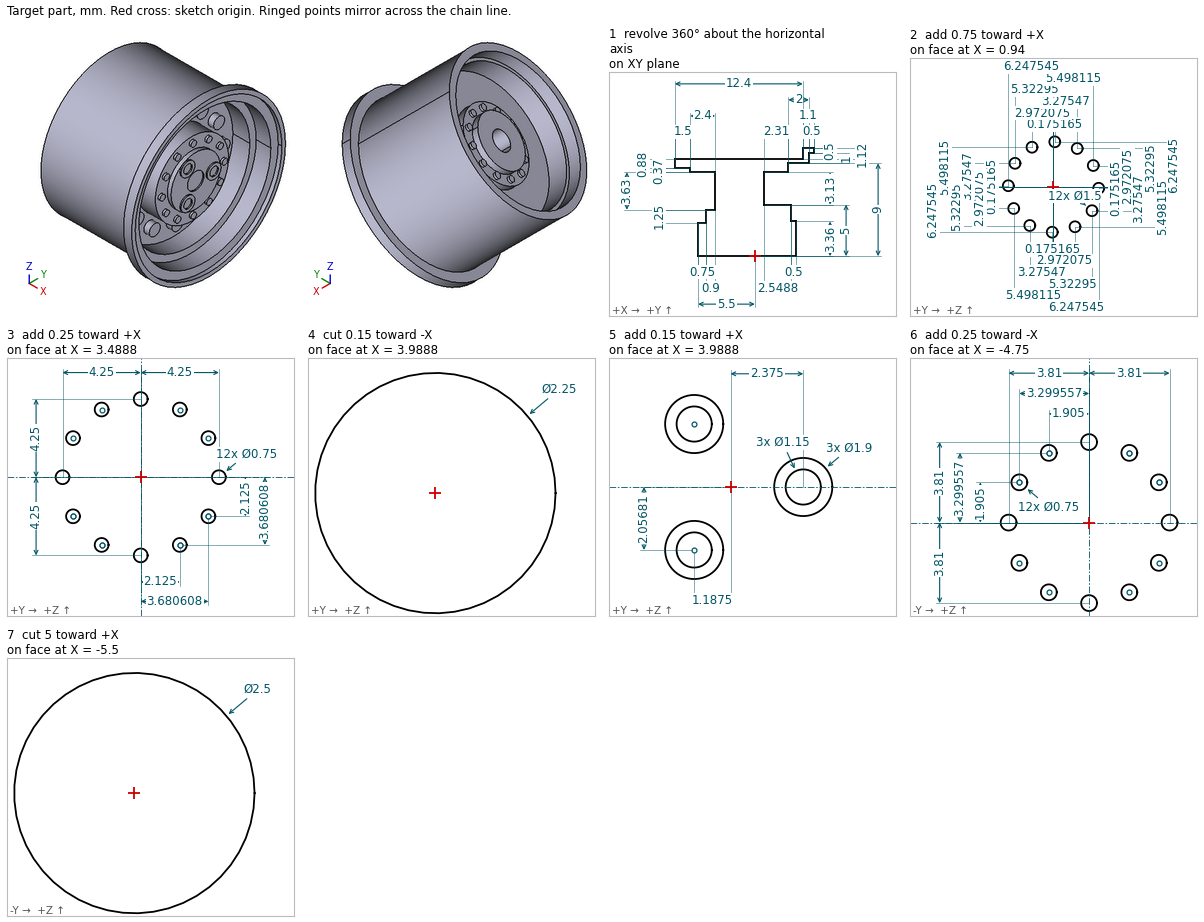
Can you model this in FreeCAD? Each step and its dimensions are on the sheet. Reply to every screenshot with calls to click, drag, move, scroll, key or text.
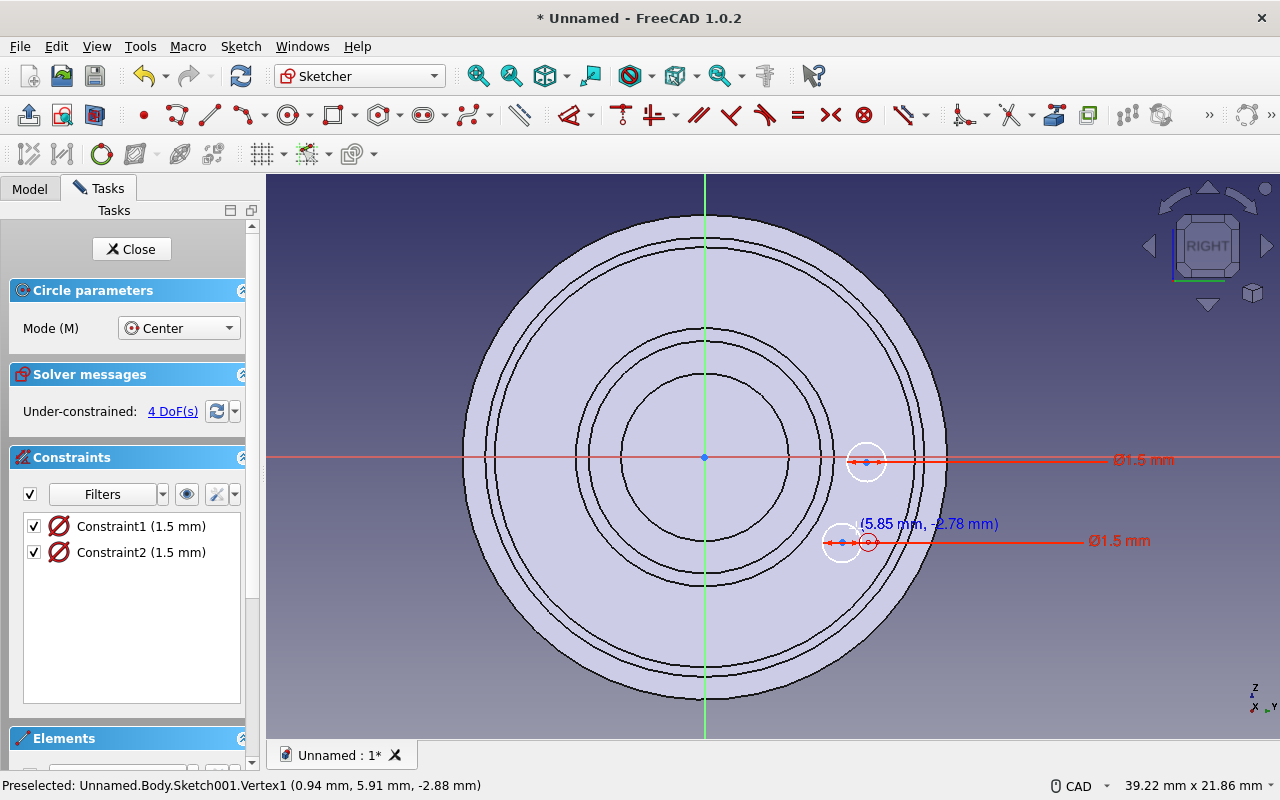
click(782, 599)
move(795, 586)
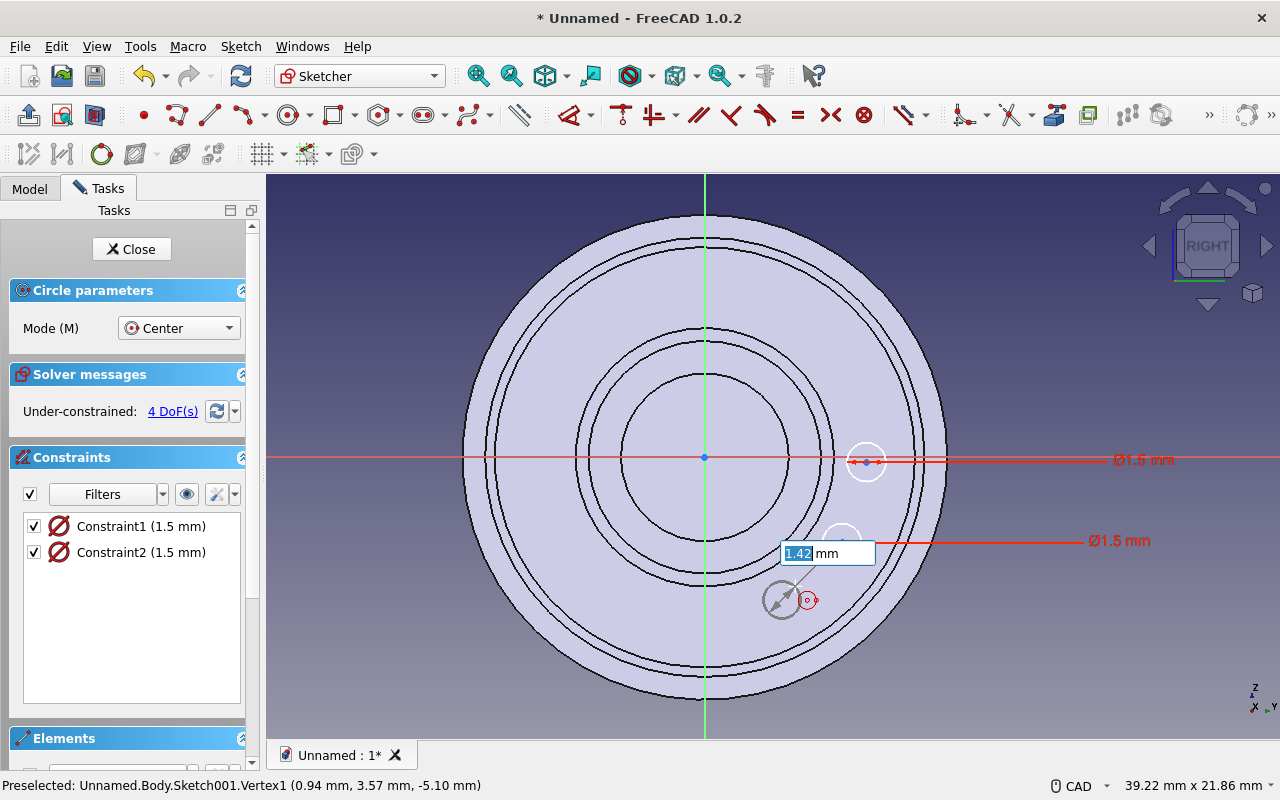
text(1.5)
key(Return)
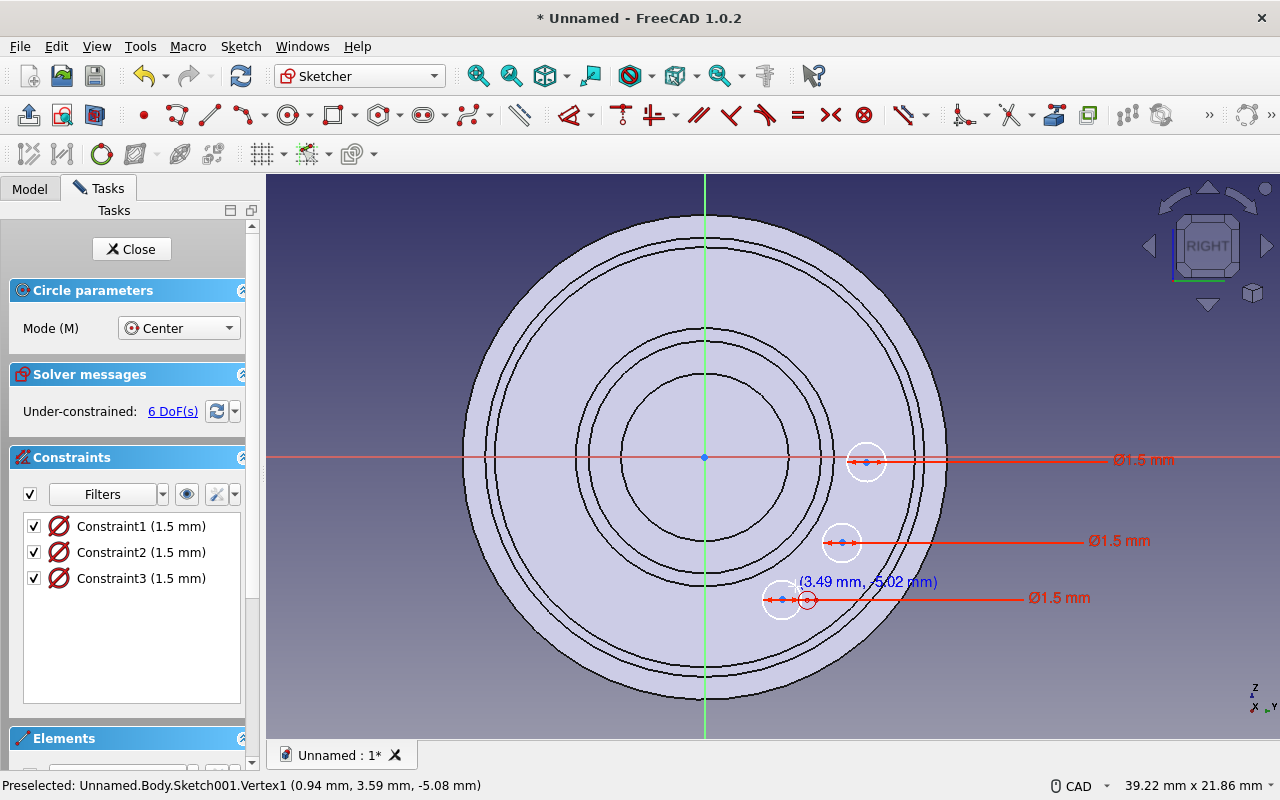
scroll(700, 619, up, 7)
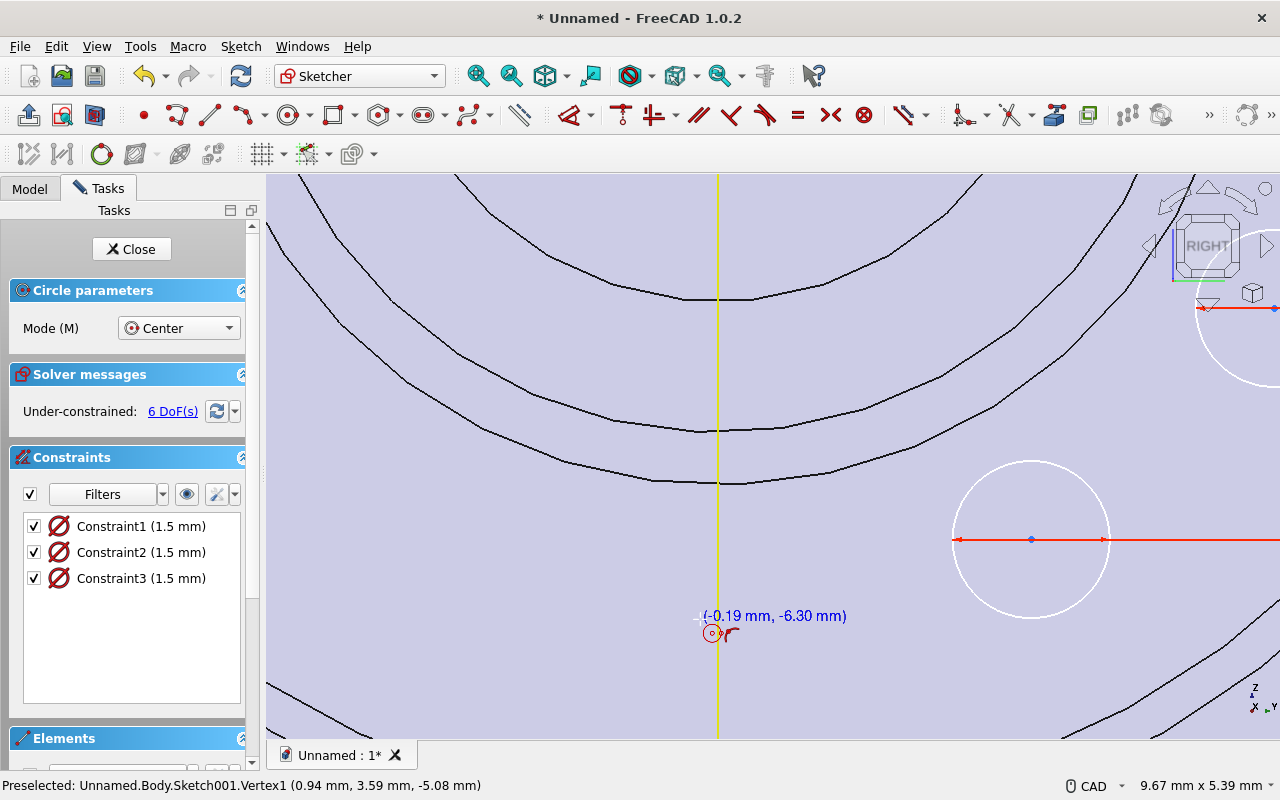
click(700, 616)
move(756, 560)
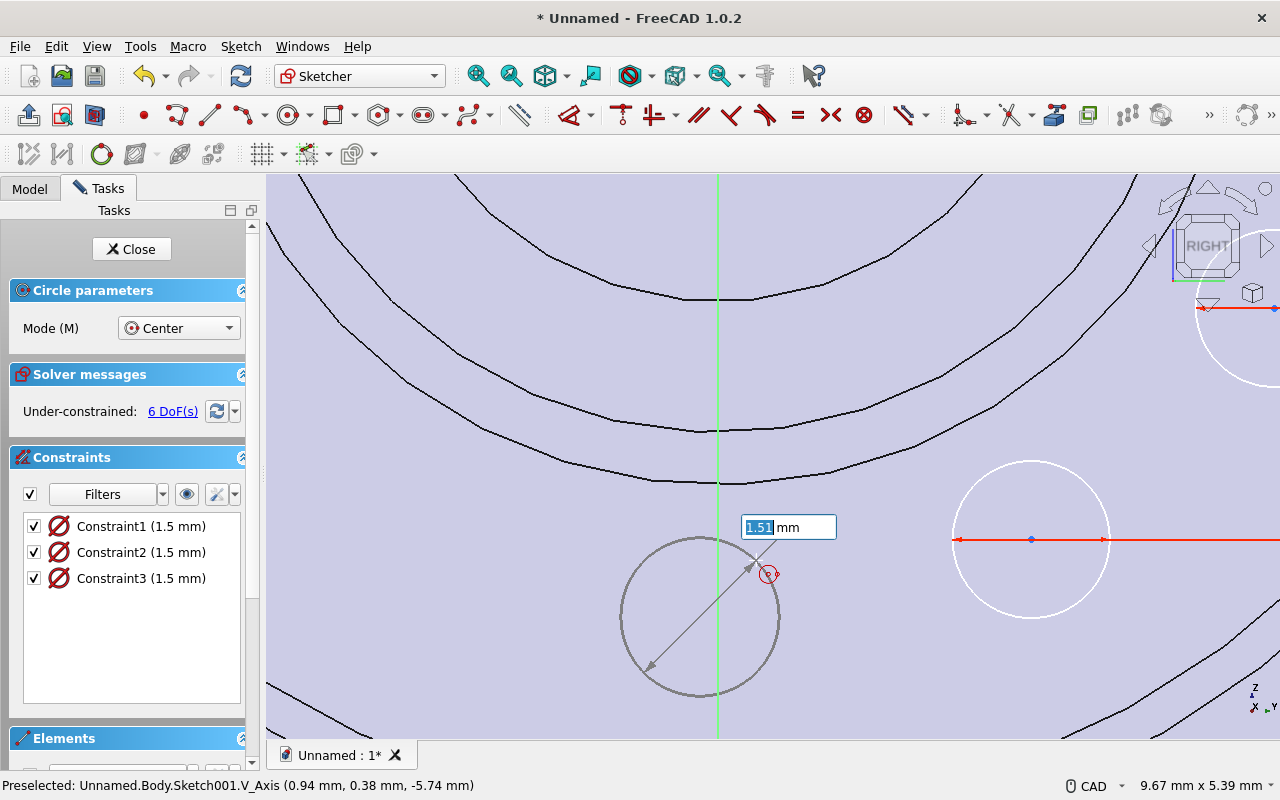
text(1.5)
key(Return)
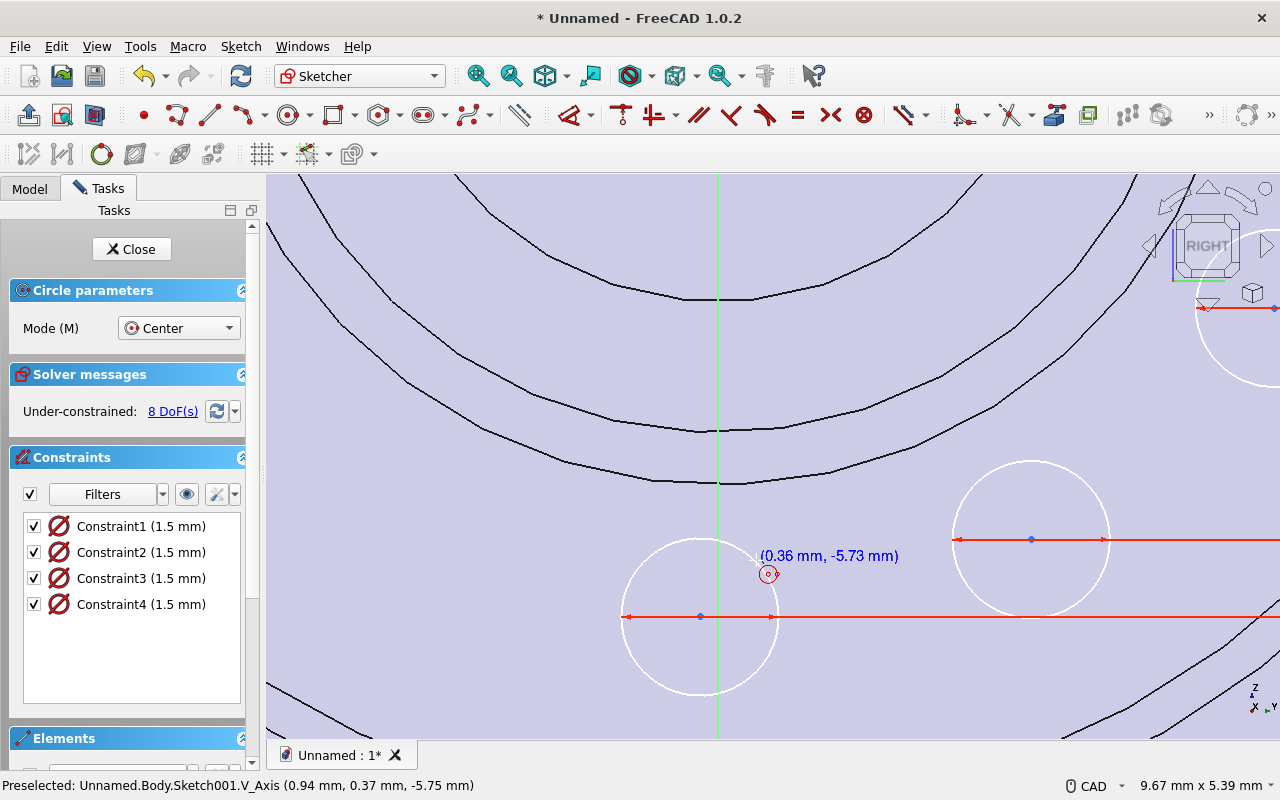
scroll(700, 619, down, 7)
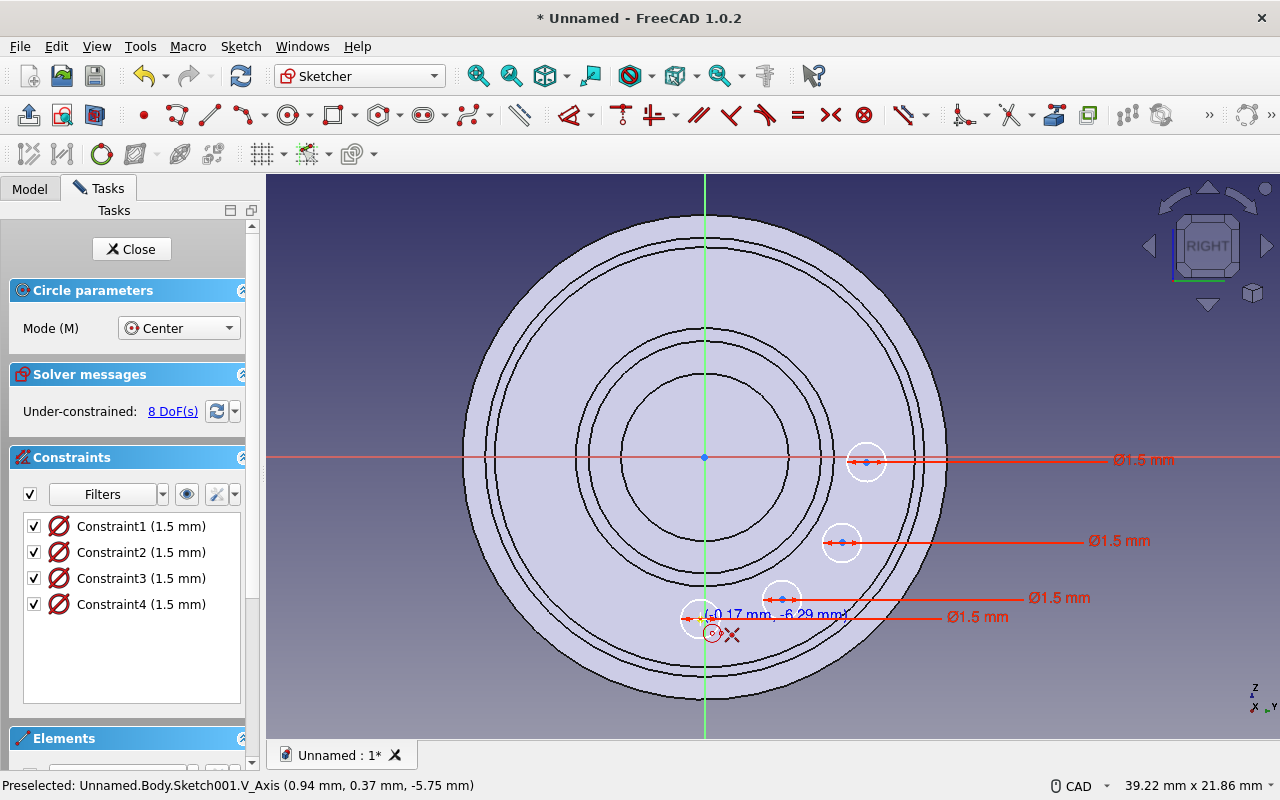
click(620, 595)
move(634, 581)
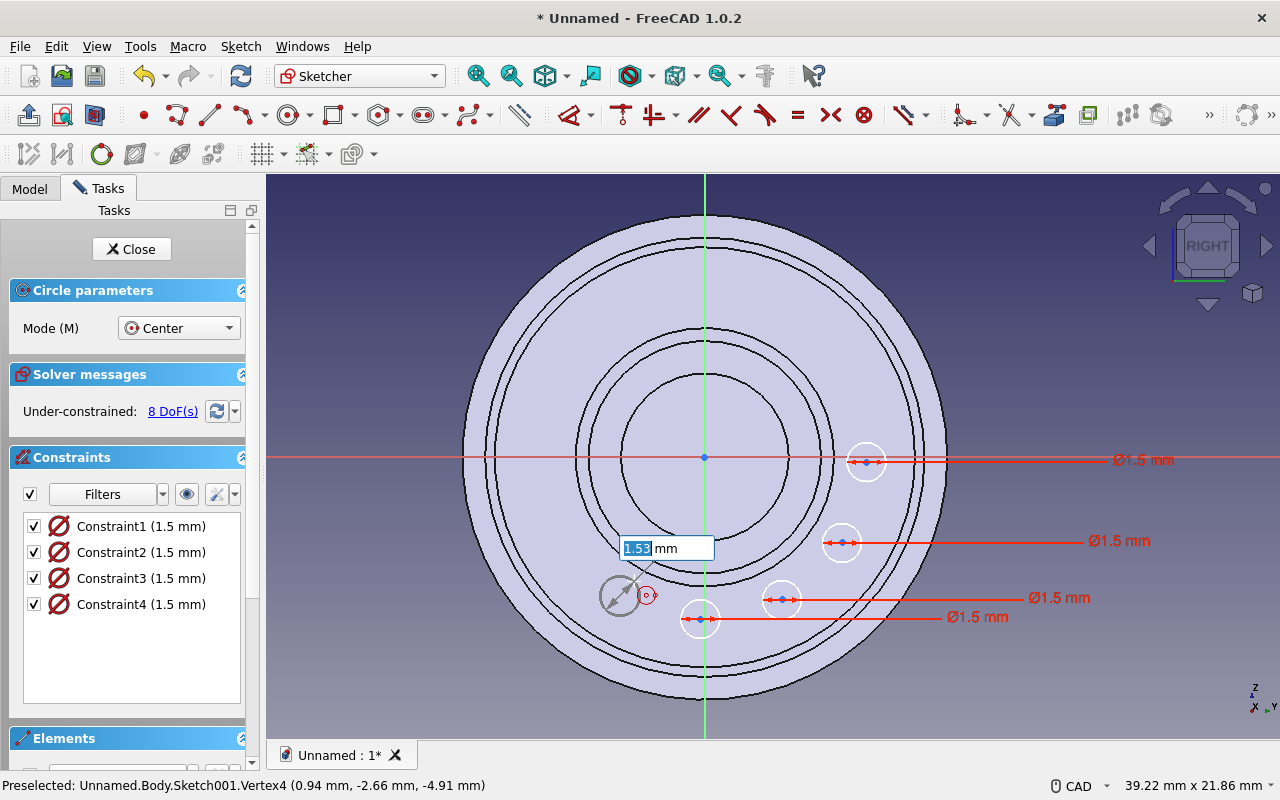
text(1.5)
key(Return)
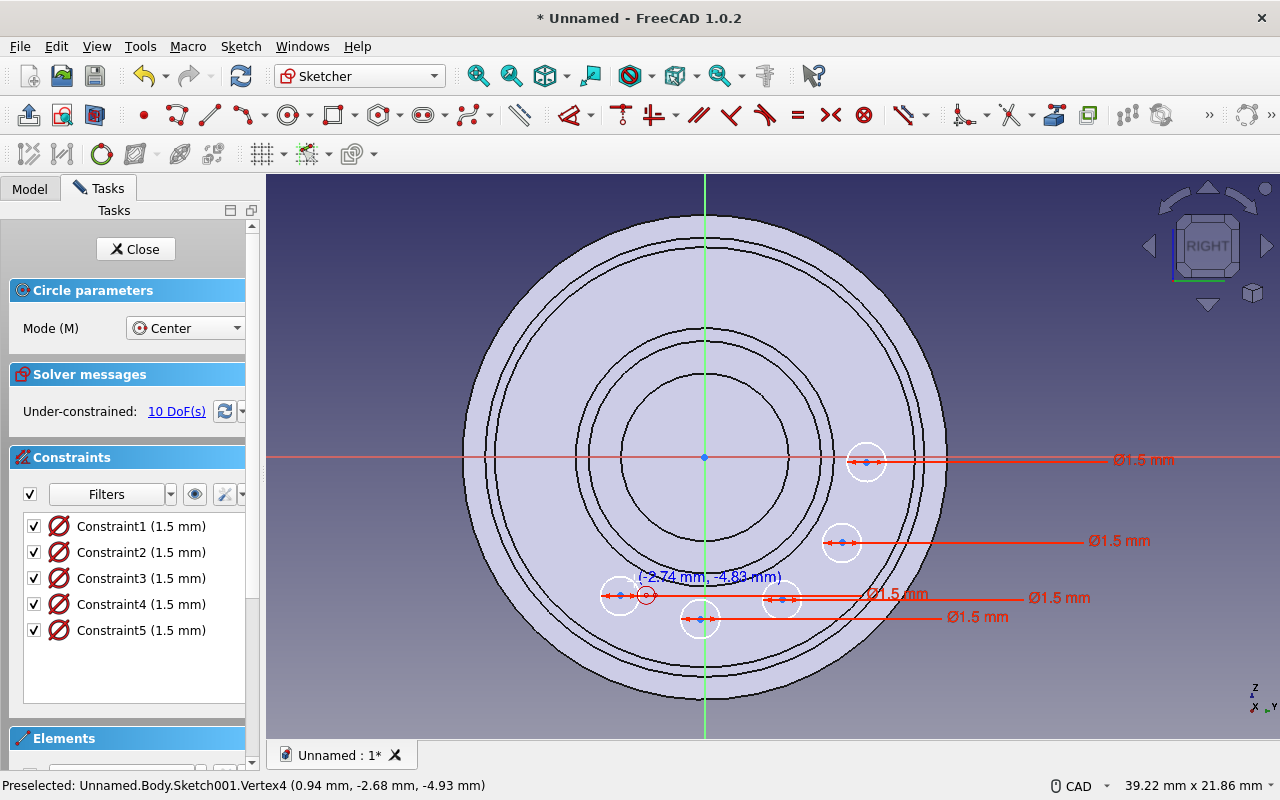
click(563, 534)
move(576, 520)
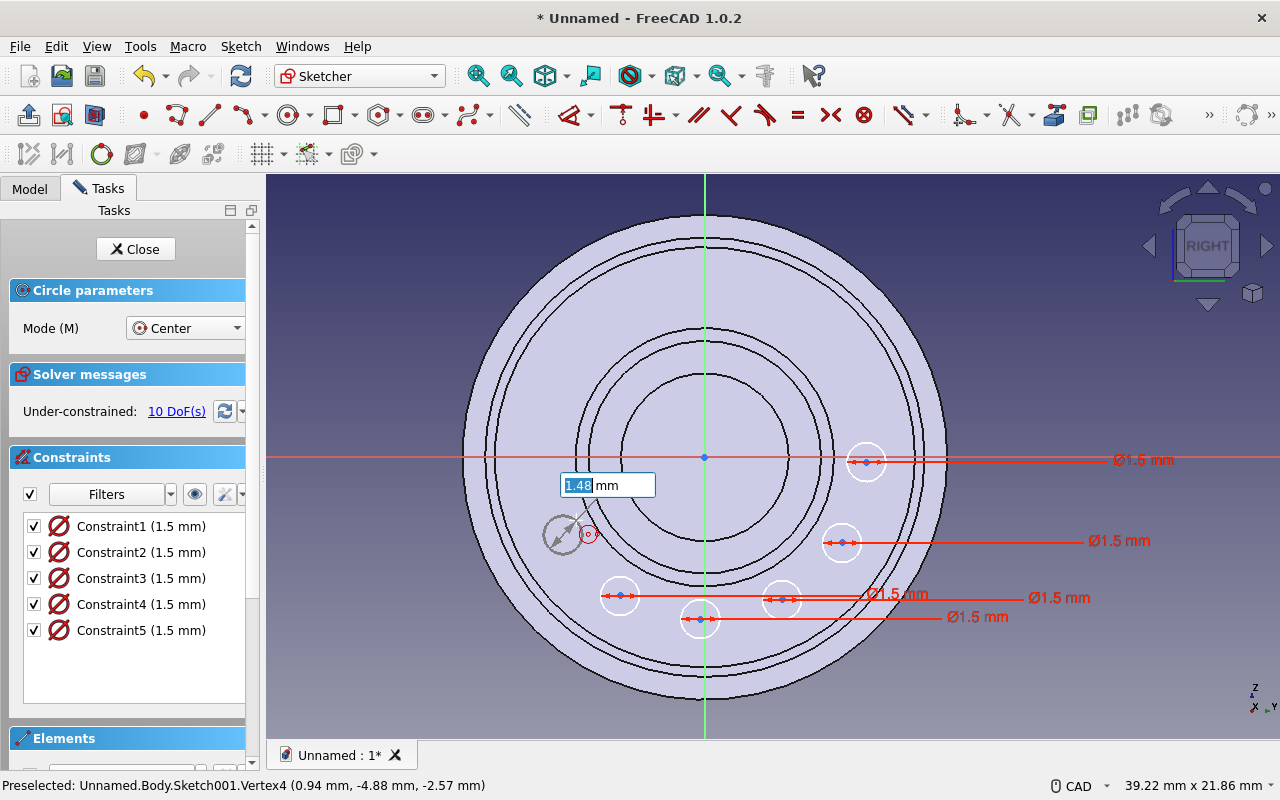
text(1.5)
key(Return)